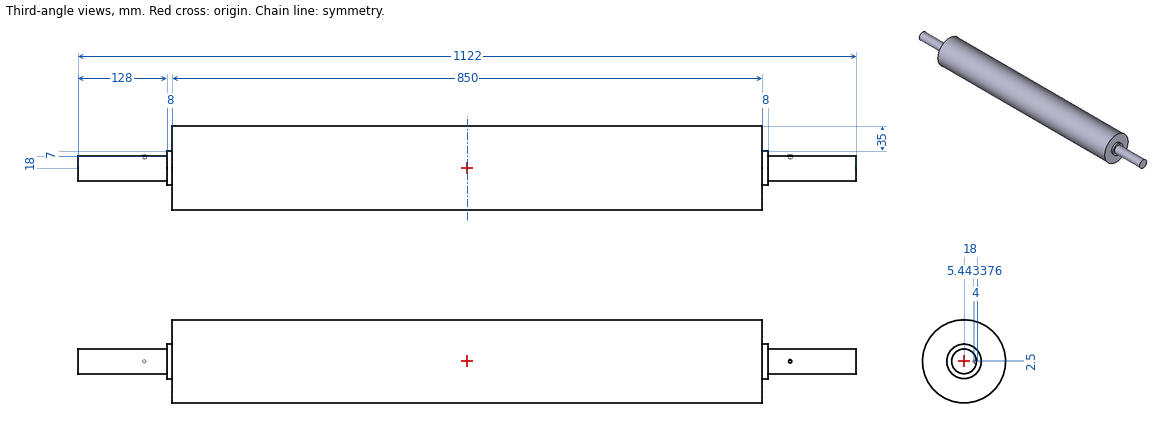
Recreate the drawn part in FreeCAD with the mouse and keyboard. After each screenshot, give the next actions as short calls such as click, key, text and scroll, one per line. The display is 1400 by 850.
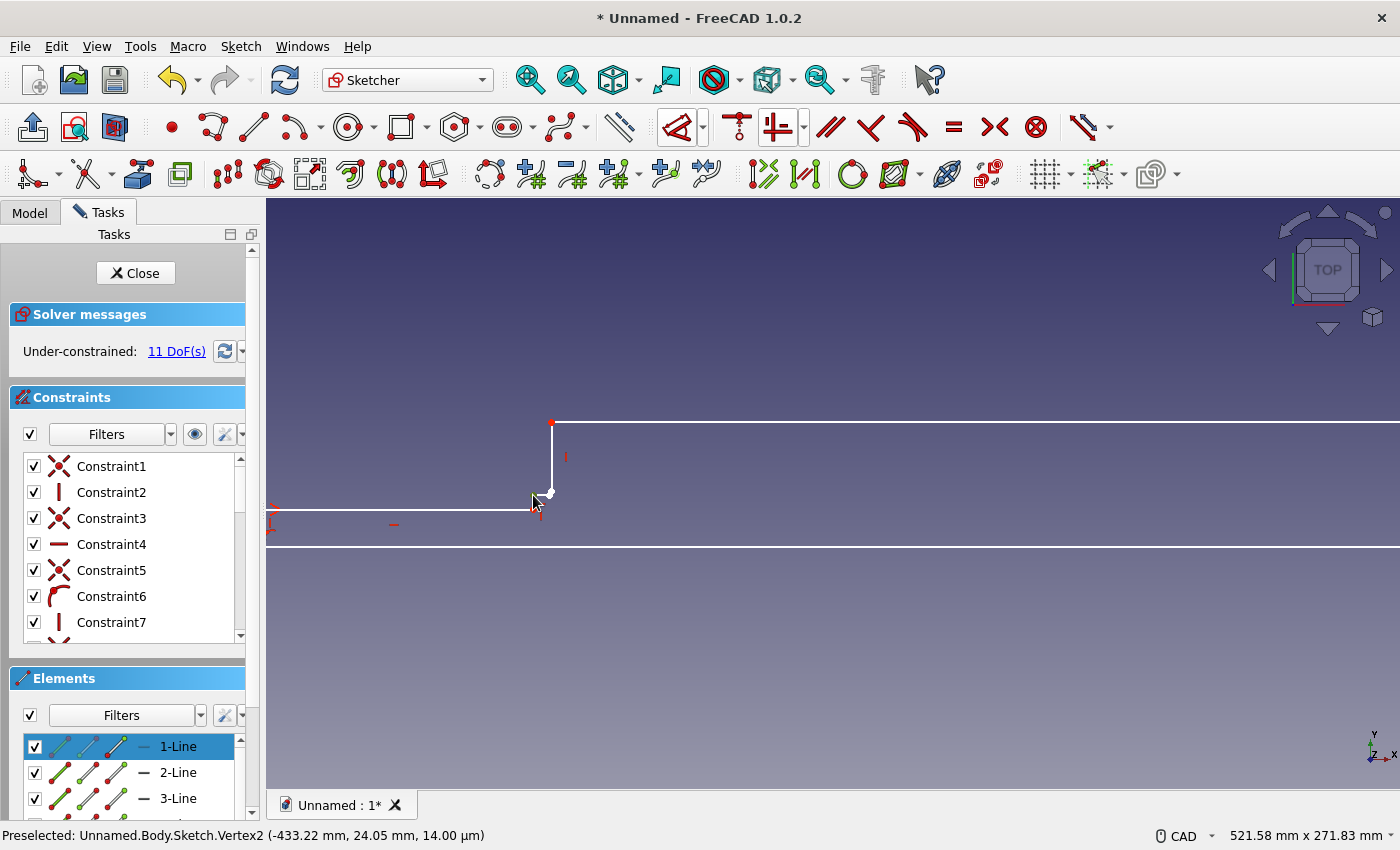
scroll(532, 497, down, 7)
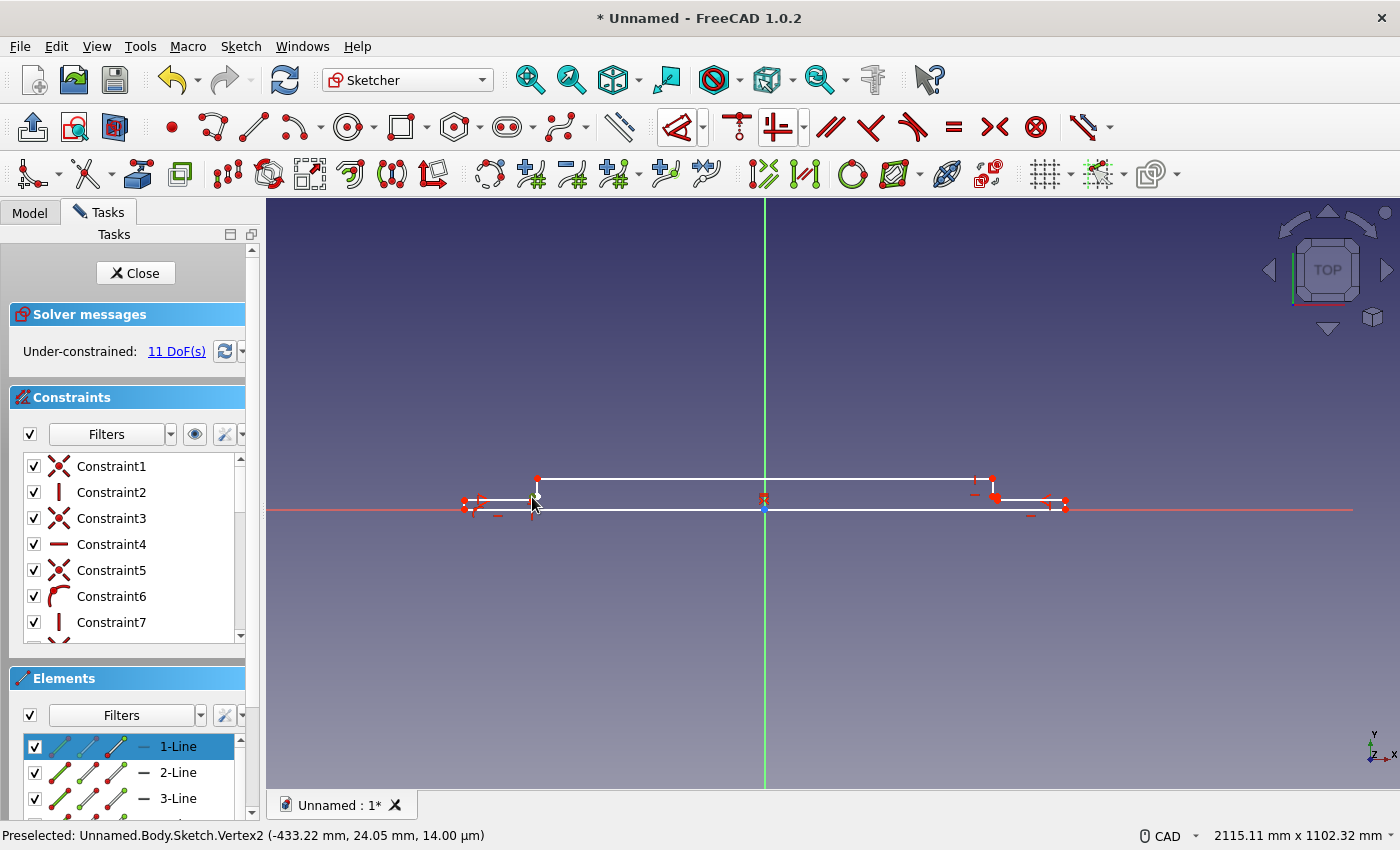
scroll(997, 497, up, 6)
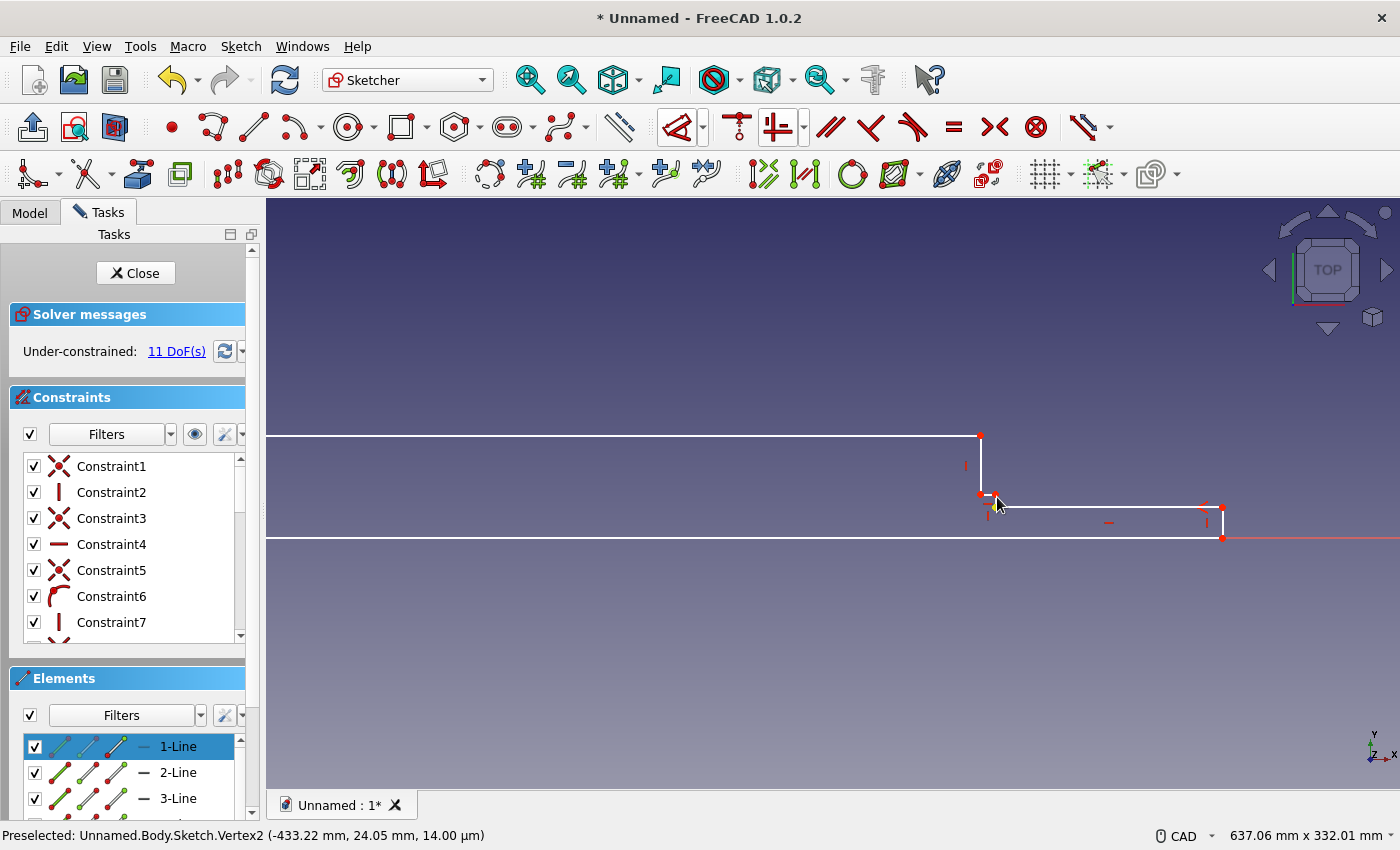
click(996, 495)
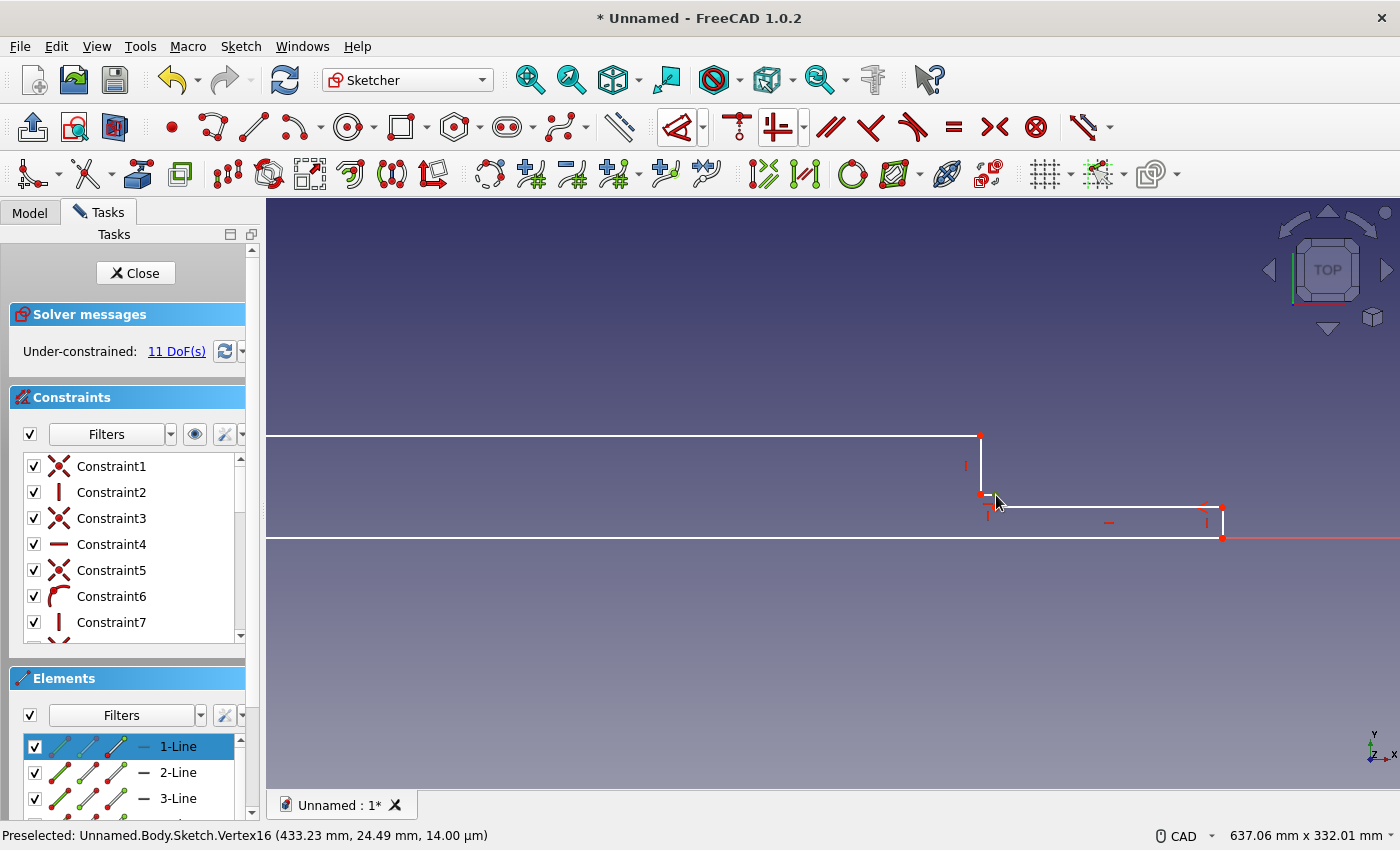
scroll(997, 497, down, 6)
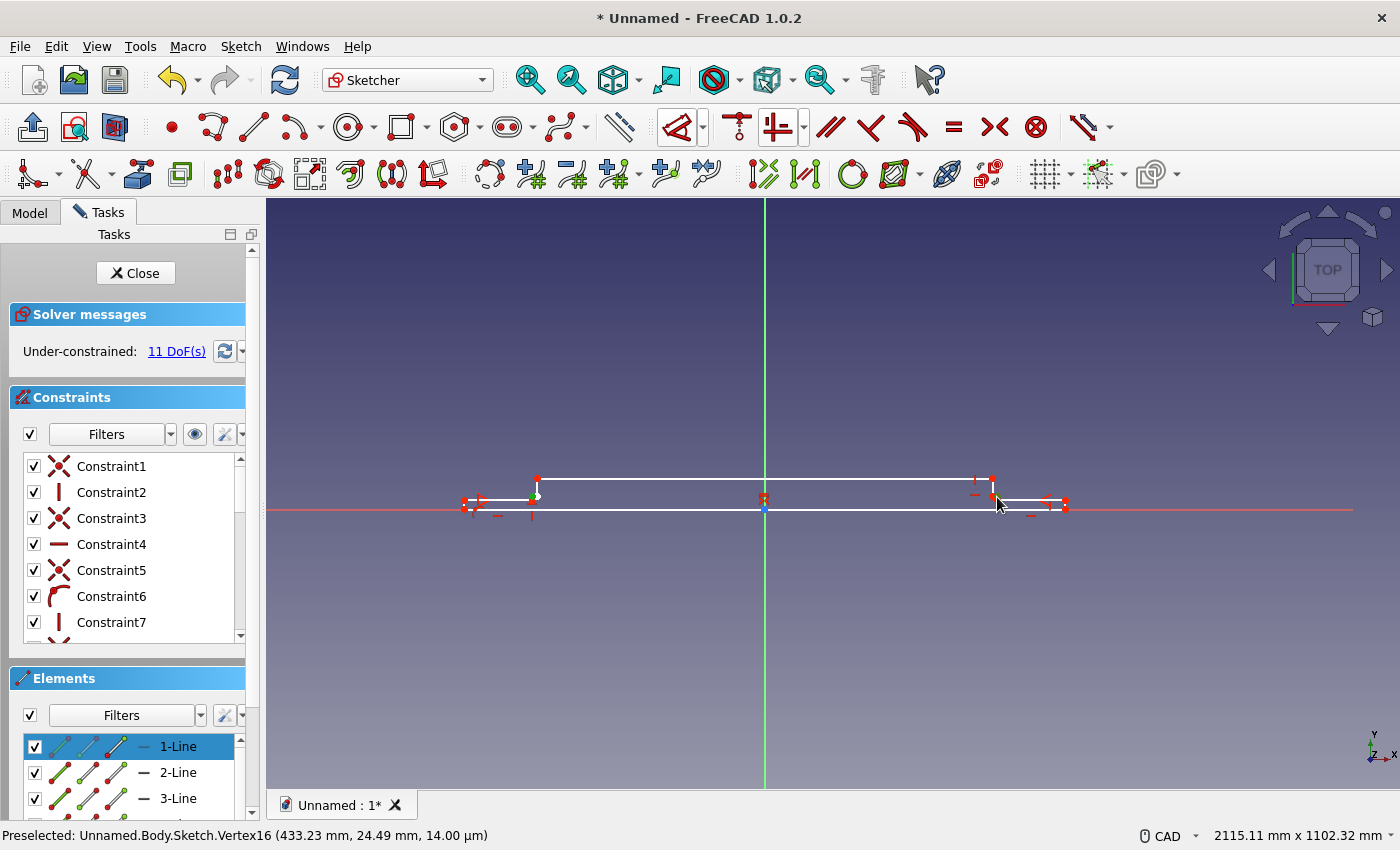
click(765, 723)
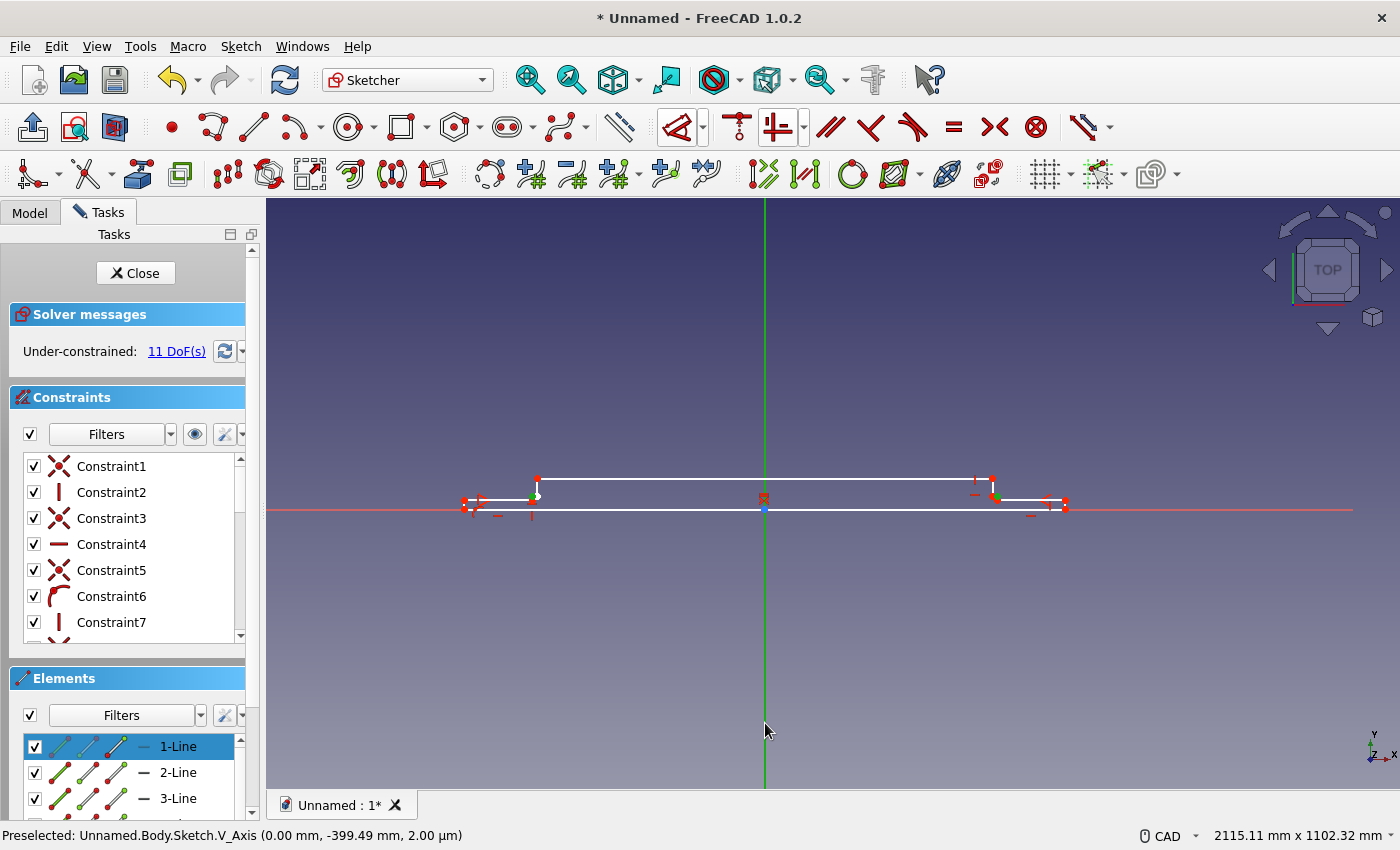
click(995, 128)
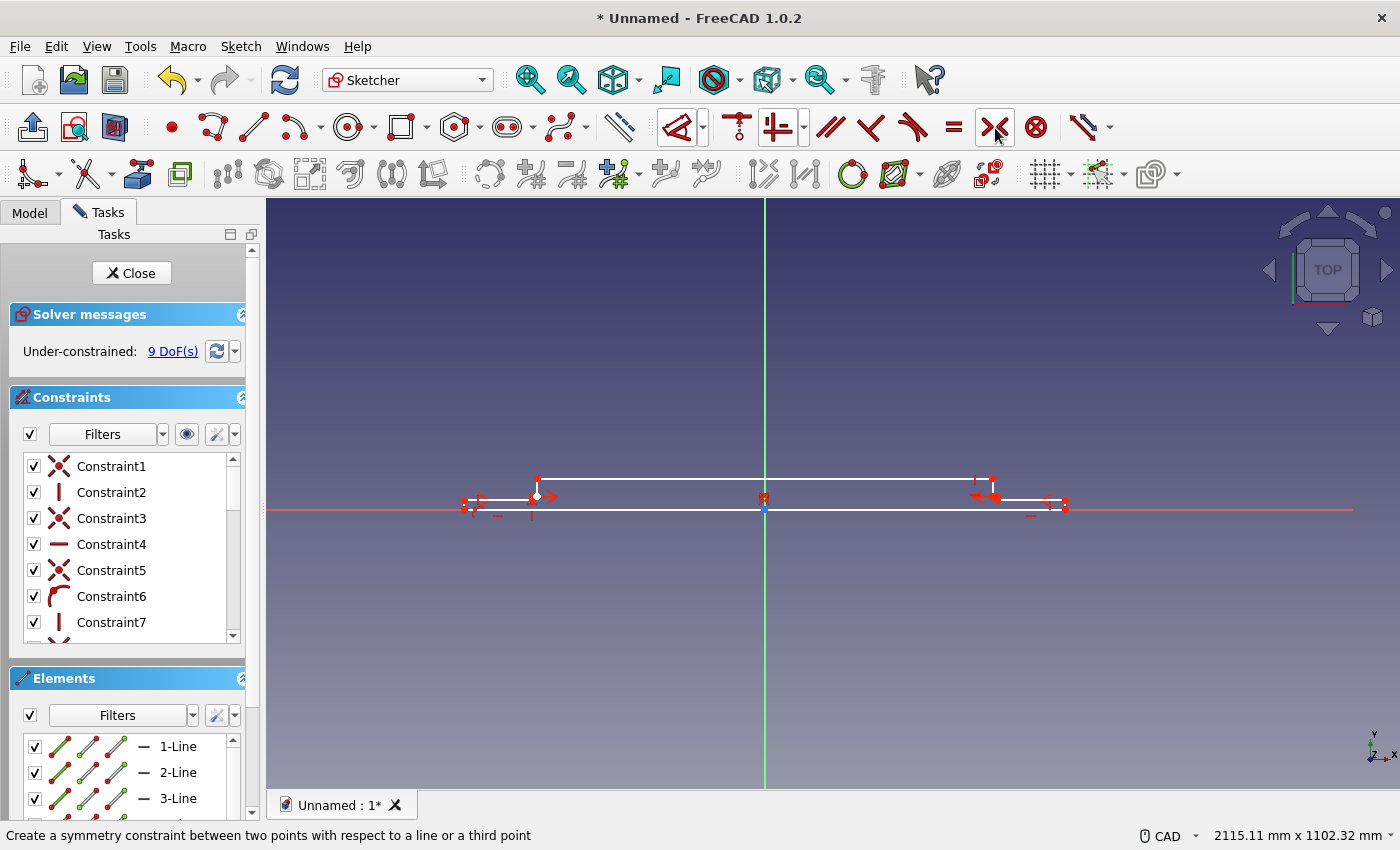
click(676, 128)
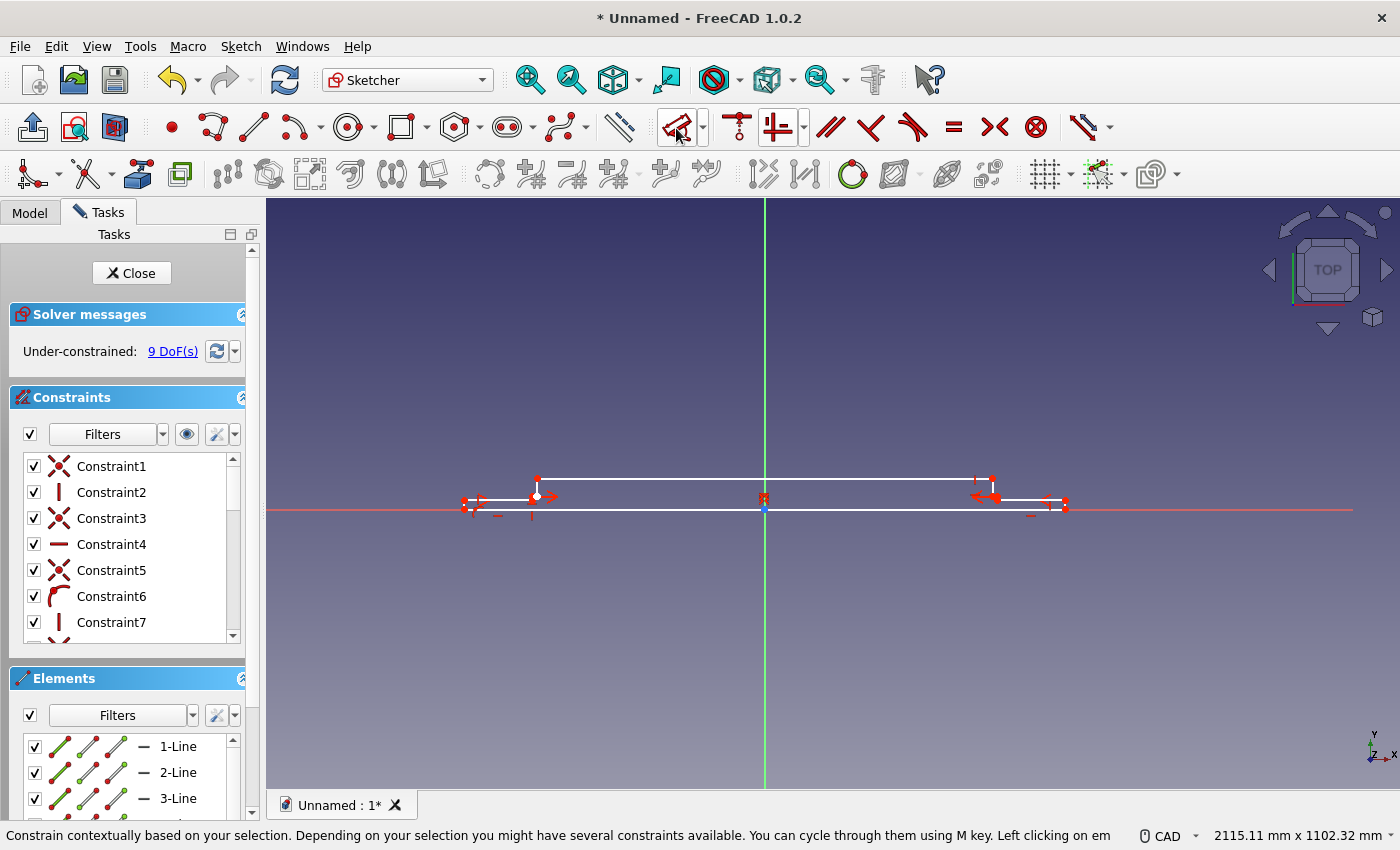
scroll(535, 497, up, 12)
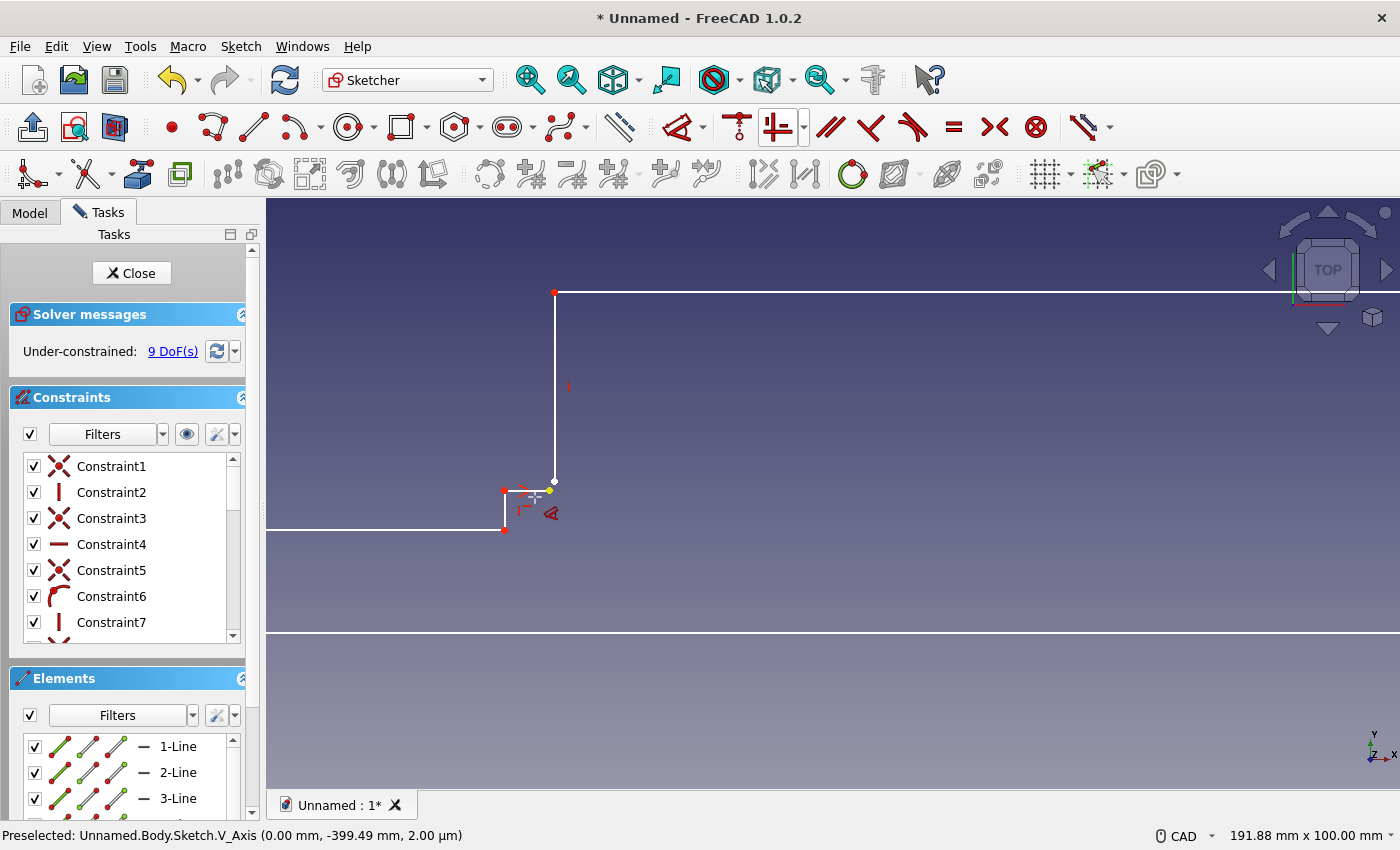
click(527, 491)
click(527, 525)